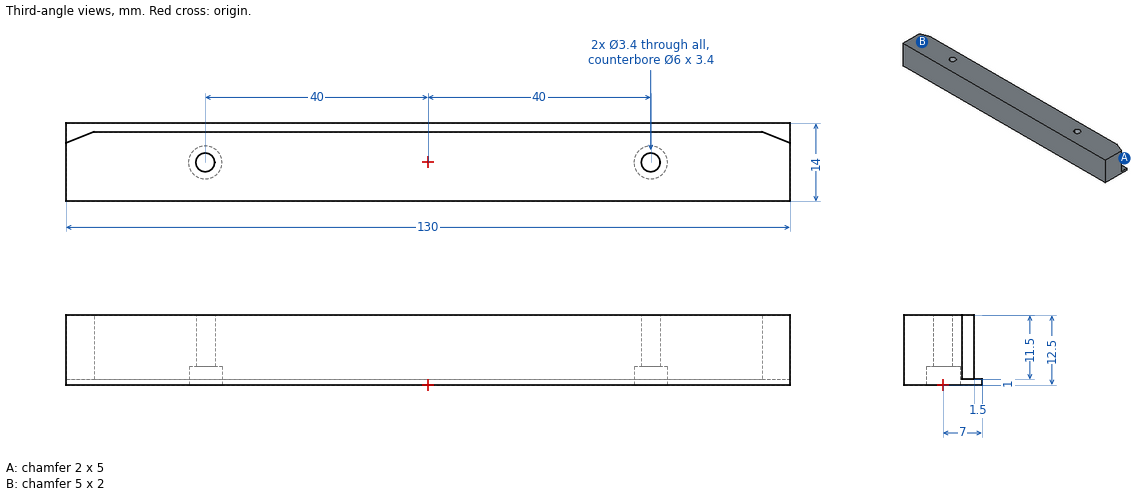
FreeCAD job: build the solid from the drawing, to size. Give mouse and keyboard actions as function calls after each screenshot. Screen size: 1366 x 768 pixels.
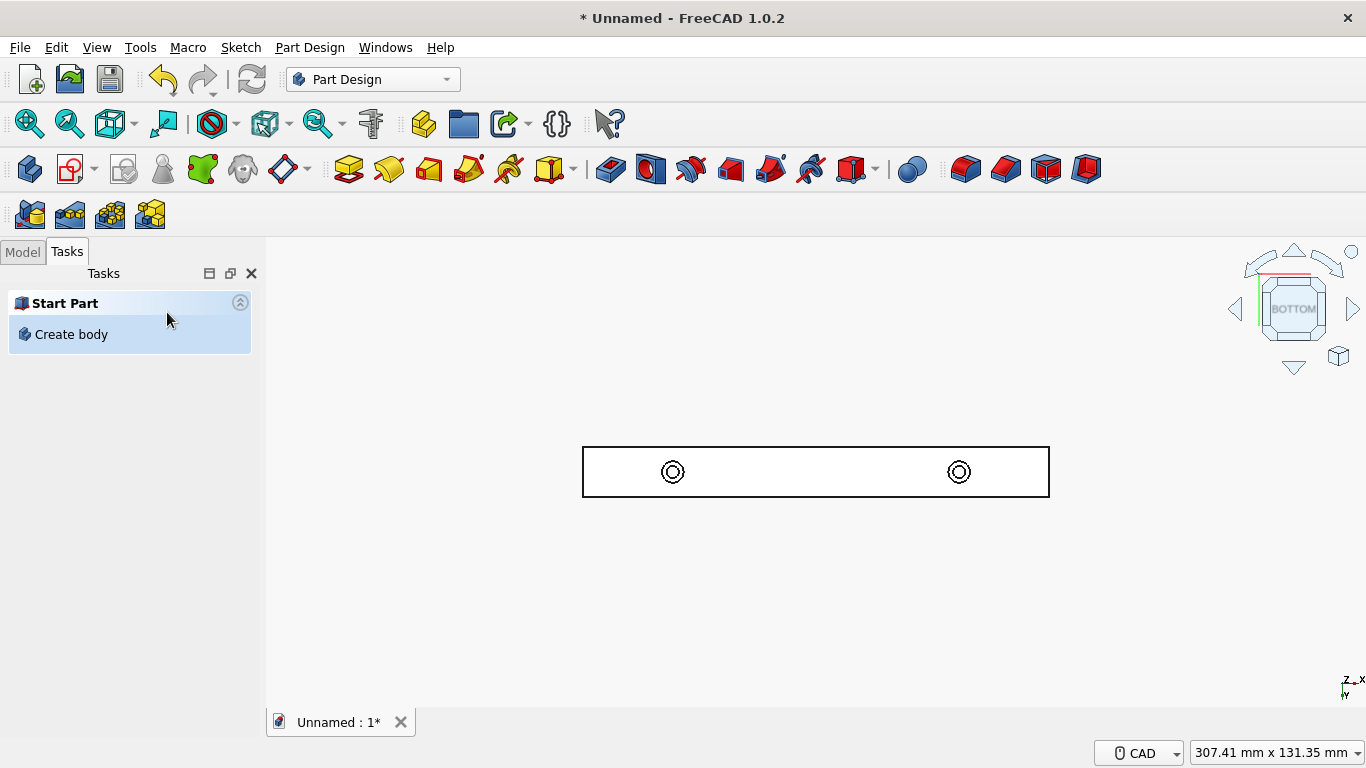
key(0)